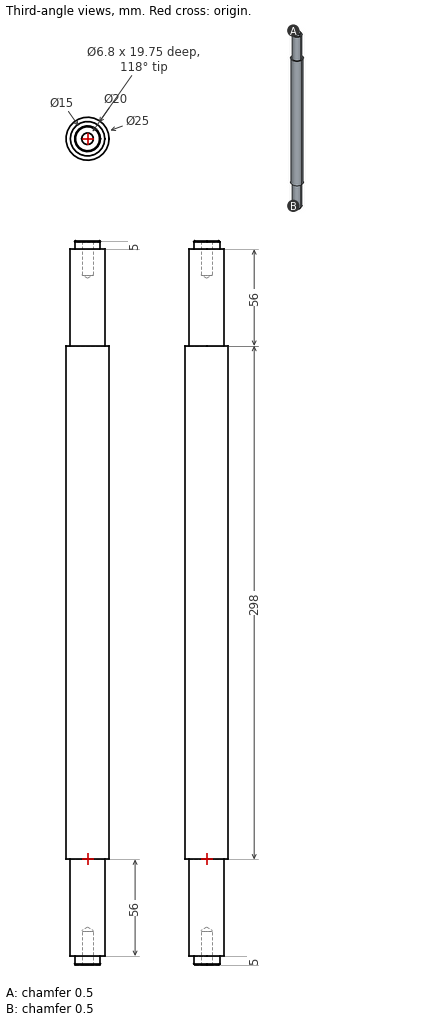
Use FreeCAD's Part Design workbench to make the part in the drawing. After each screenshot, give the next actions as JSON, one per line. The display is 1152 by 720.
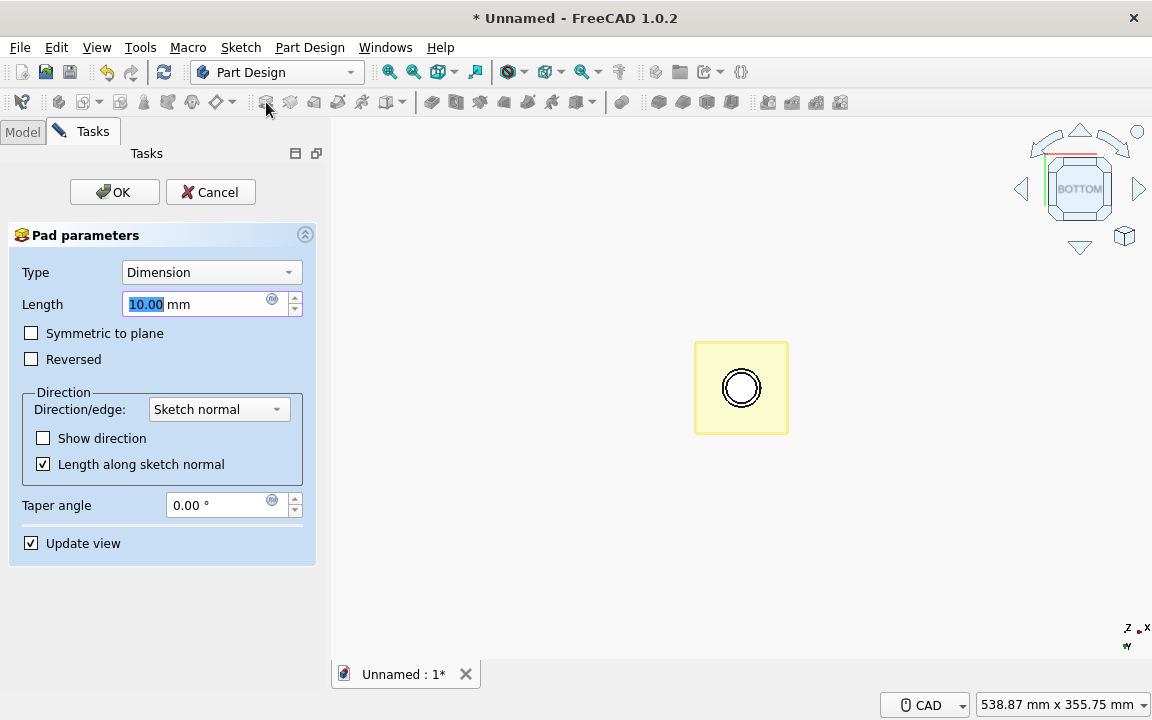
{"action": "type", "text": "56"}
{"action": "key", "text": "Tab"}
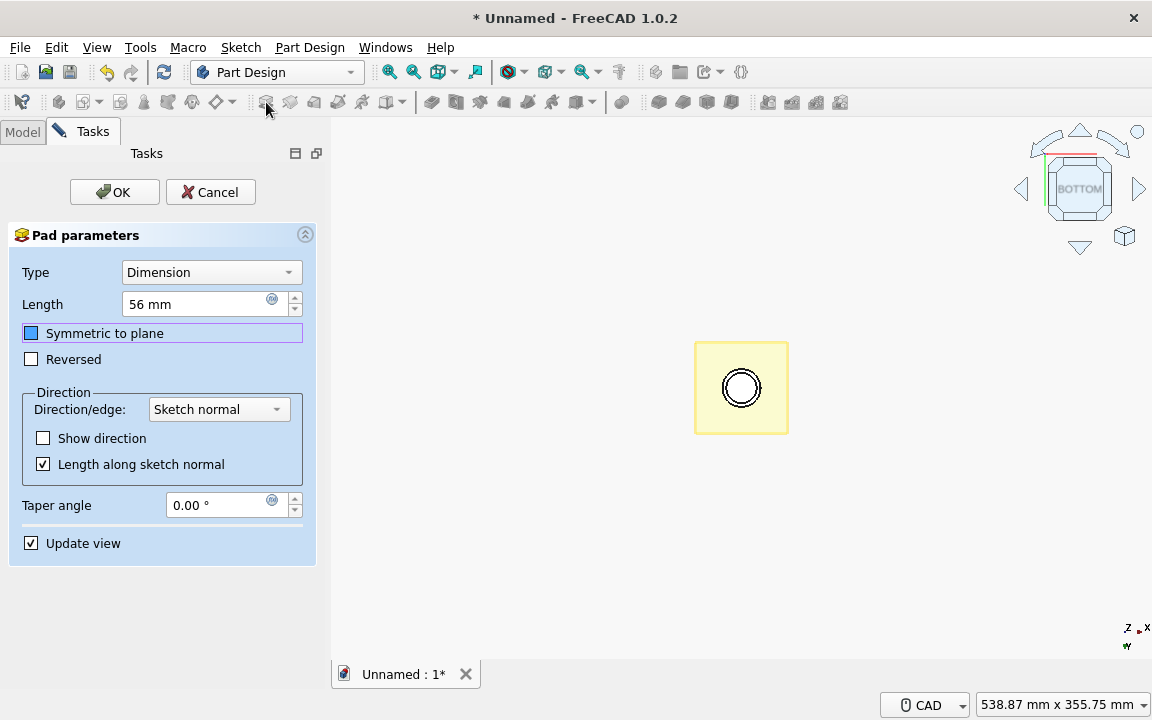
{"action": "left_click", "coordinate": [30, 359]}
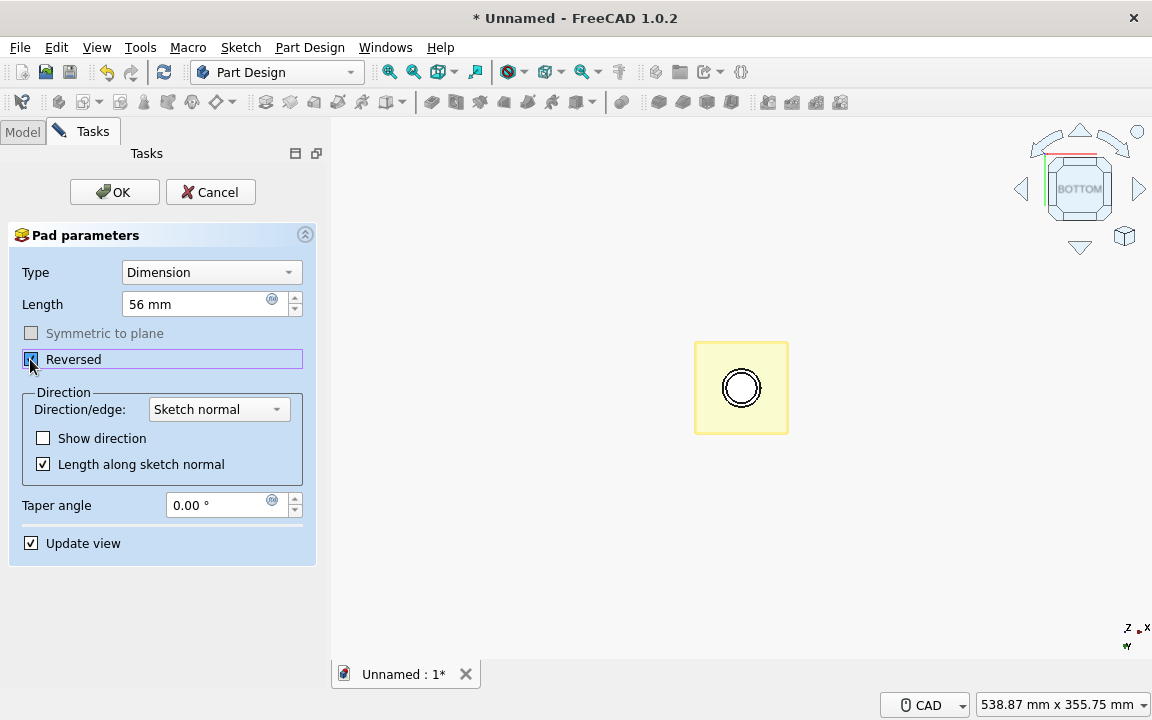
{"action": "left_click", "coordinate": [115, 192]}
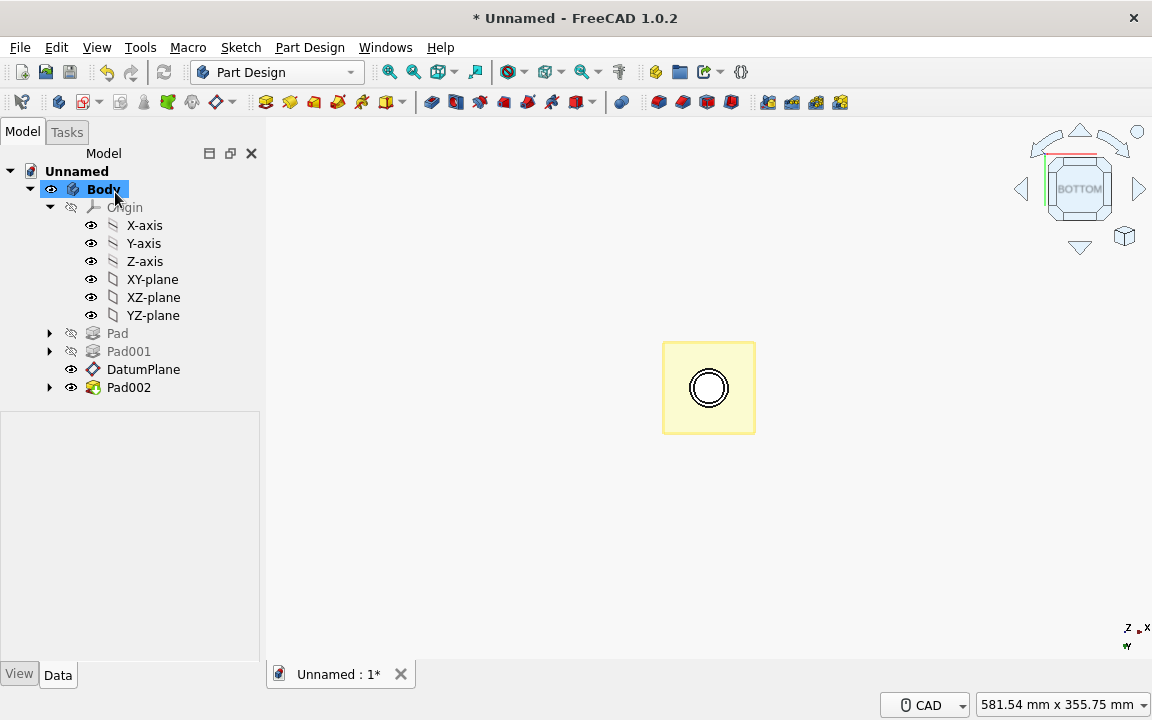
{"action": "left_click", "coordinate": [116, 369]}
{"action": "key", "text": "space"}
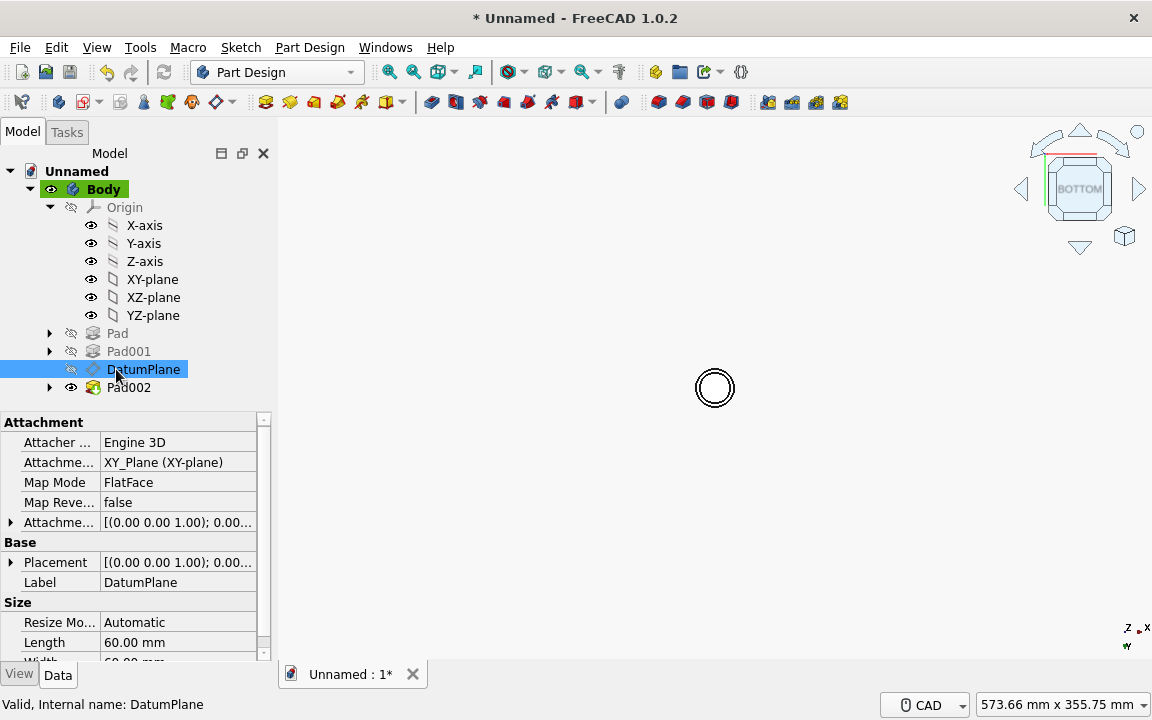
{"action": "left_click", "coordinate": [390, 72]}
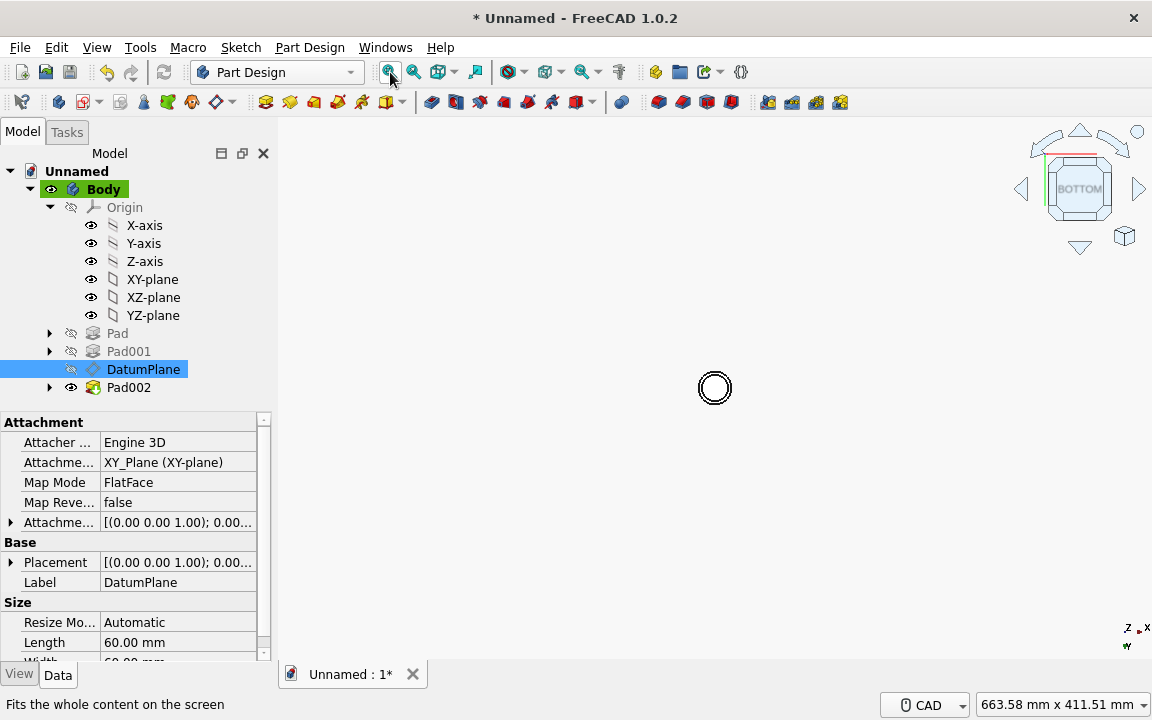
{"action": "key", "text": "0"}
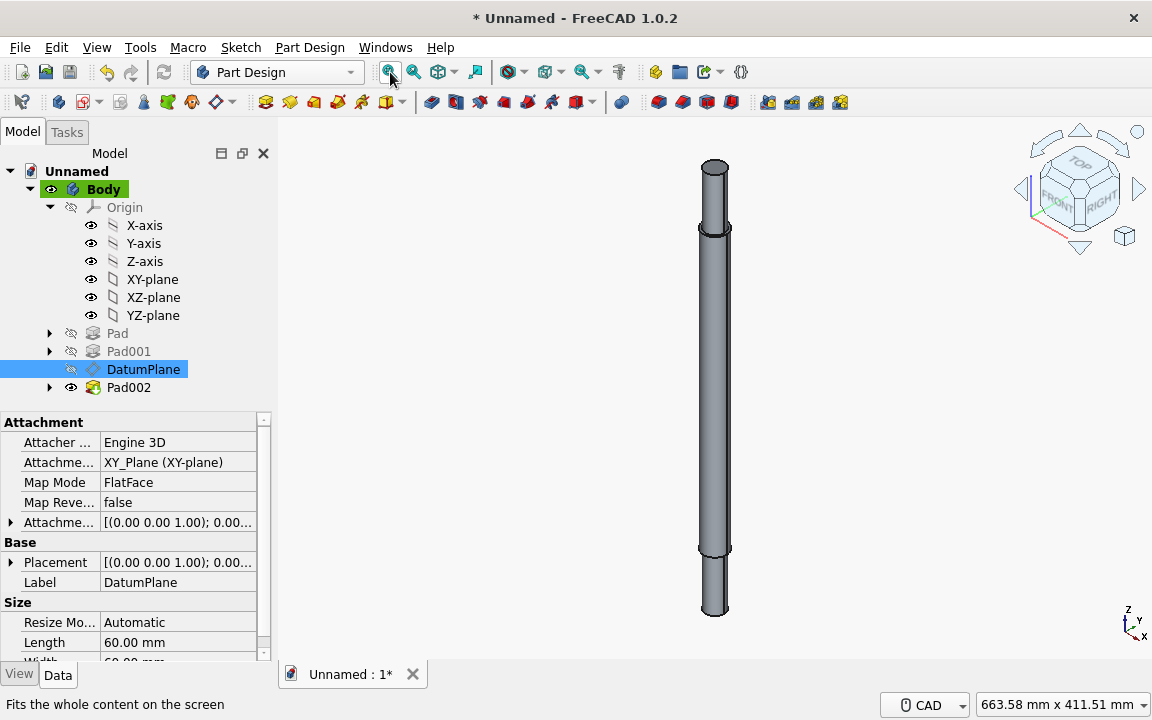
{"action": "key", "text": "2"}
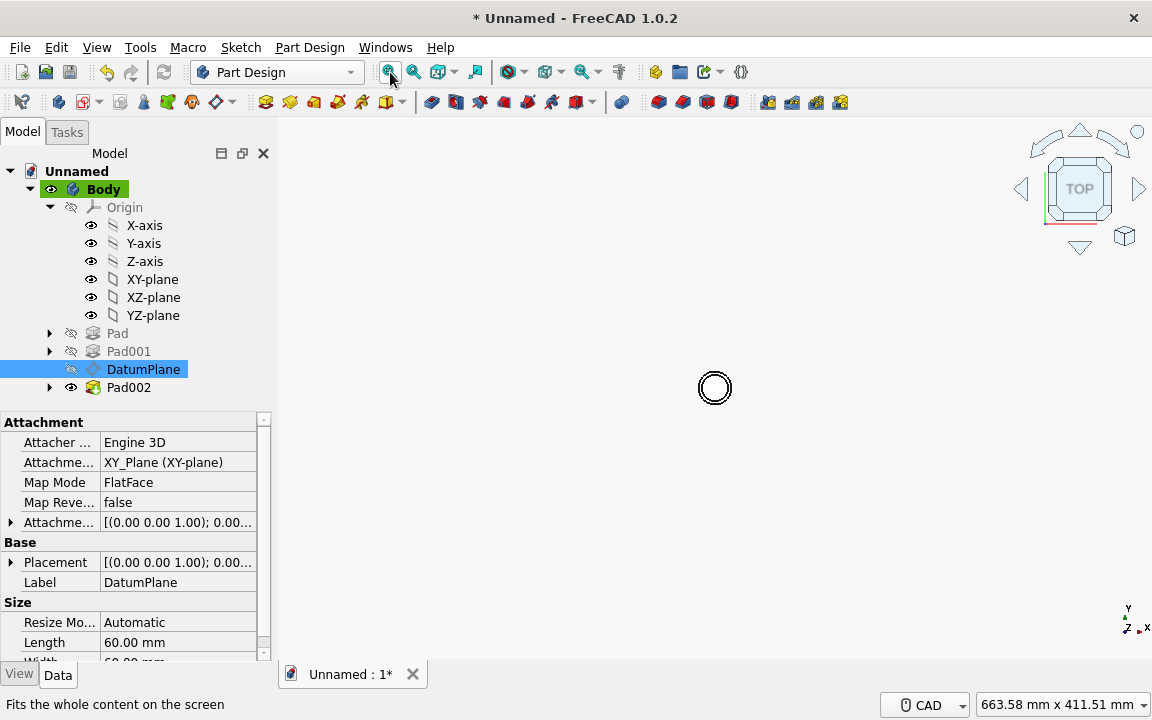
{"action": "left_click", "coordinate": [390, 72]}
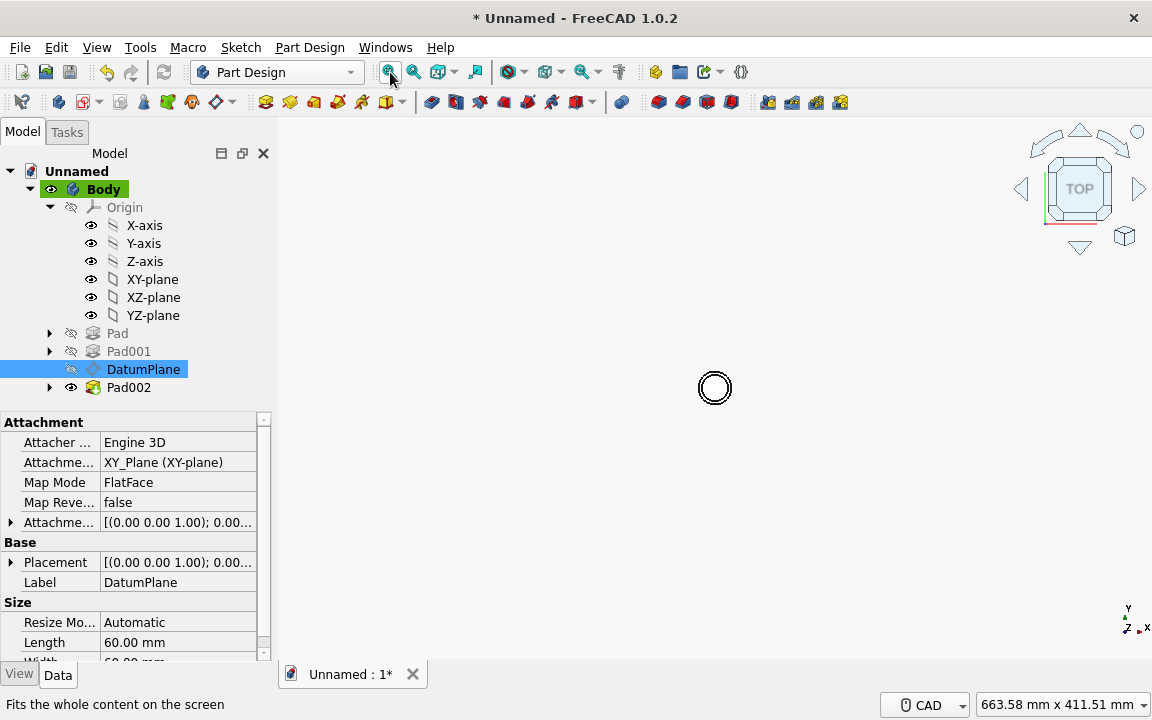
{"action": "left_click", "coordinate": [715, 387]}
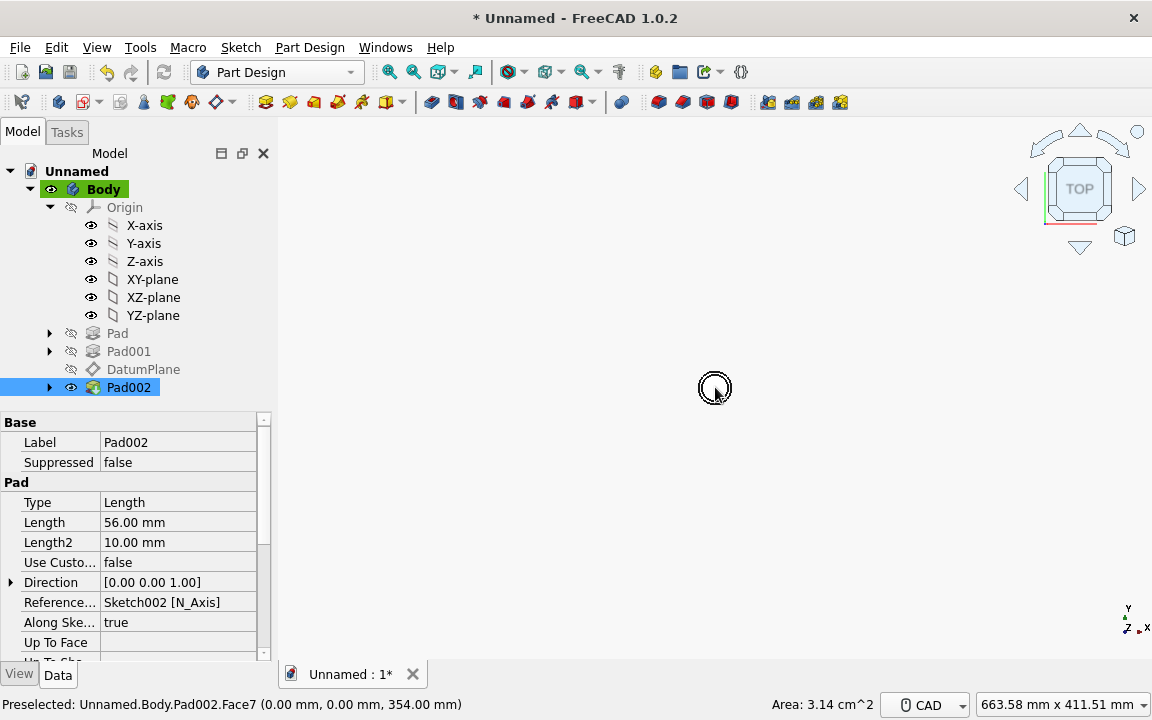
{"action": "left_click", "coordinate": [84, 102]}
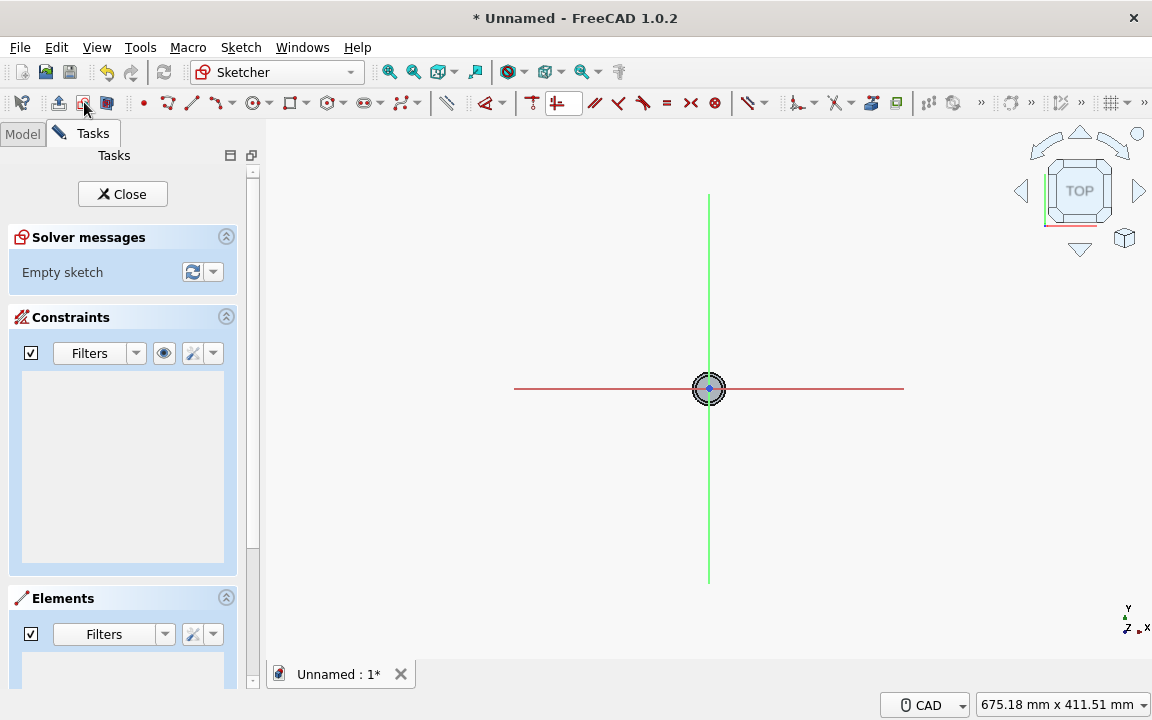
{"action": "scroll", "coordinate": [713, 389], "scroll_direction": "up", "scroll_amount": 14}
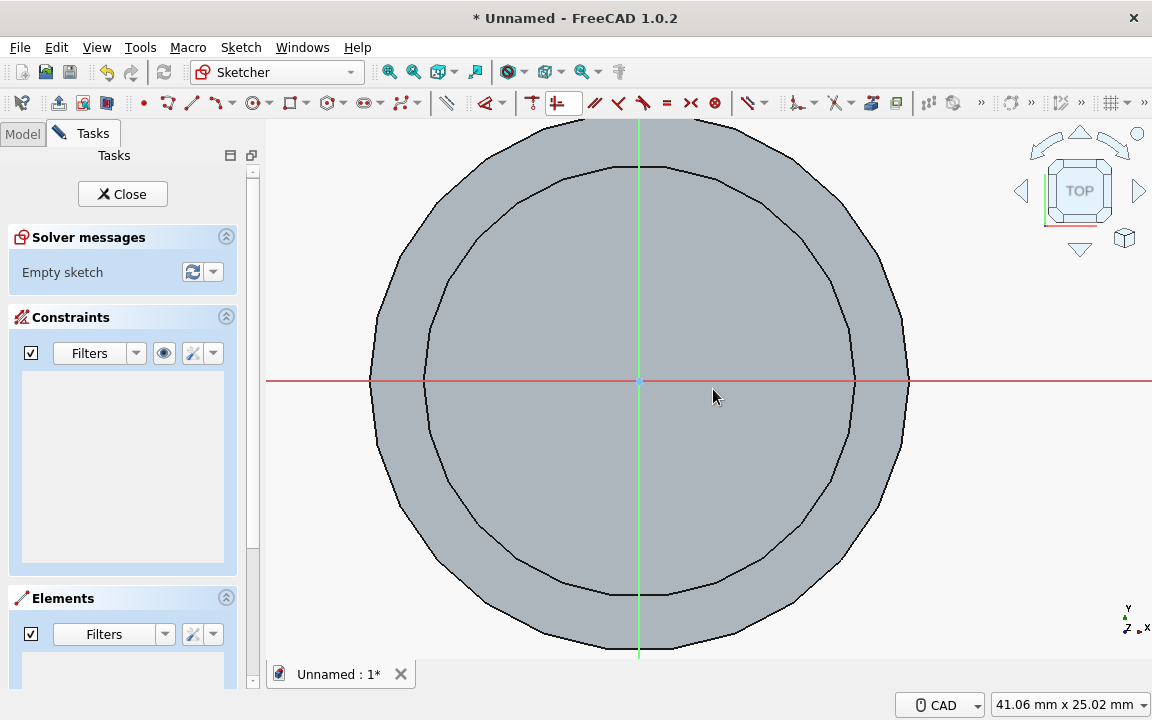
{"action": "left_click", "coordinate": [254, 104]}